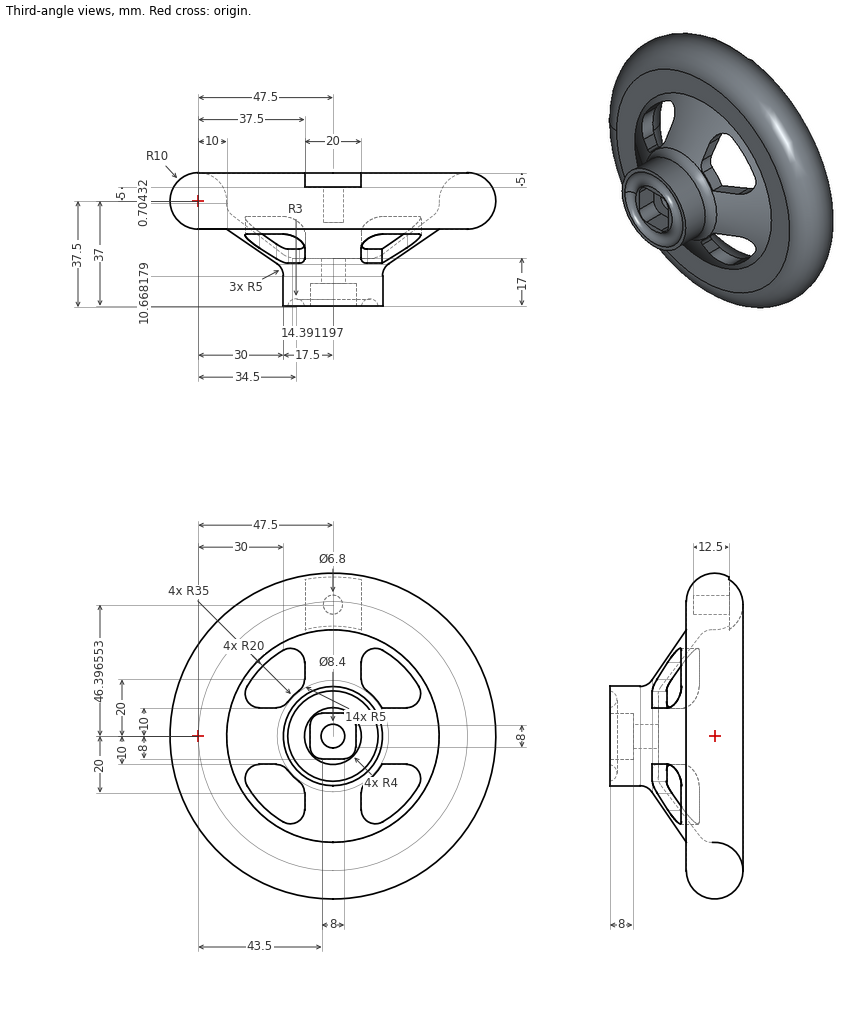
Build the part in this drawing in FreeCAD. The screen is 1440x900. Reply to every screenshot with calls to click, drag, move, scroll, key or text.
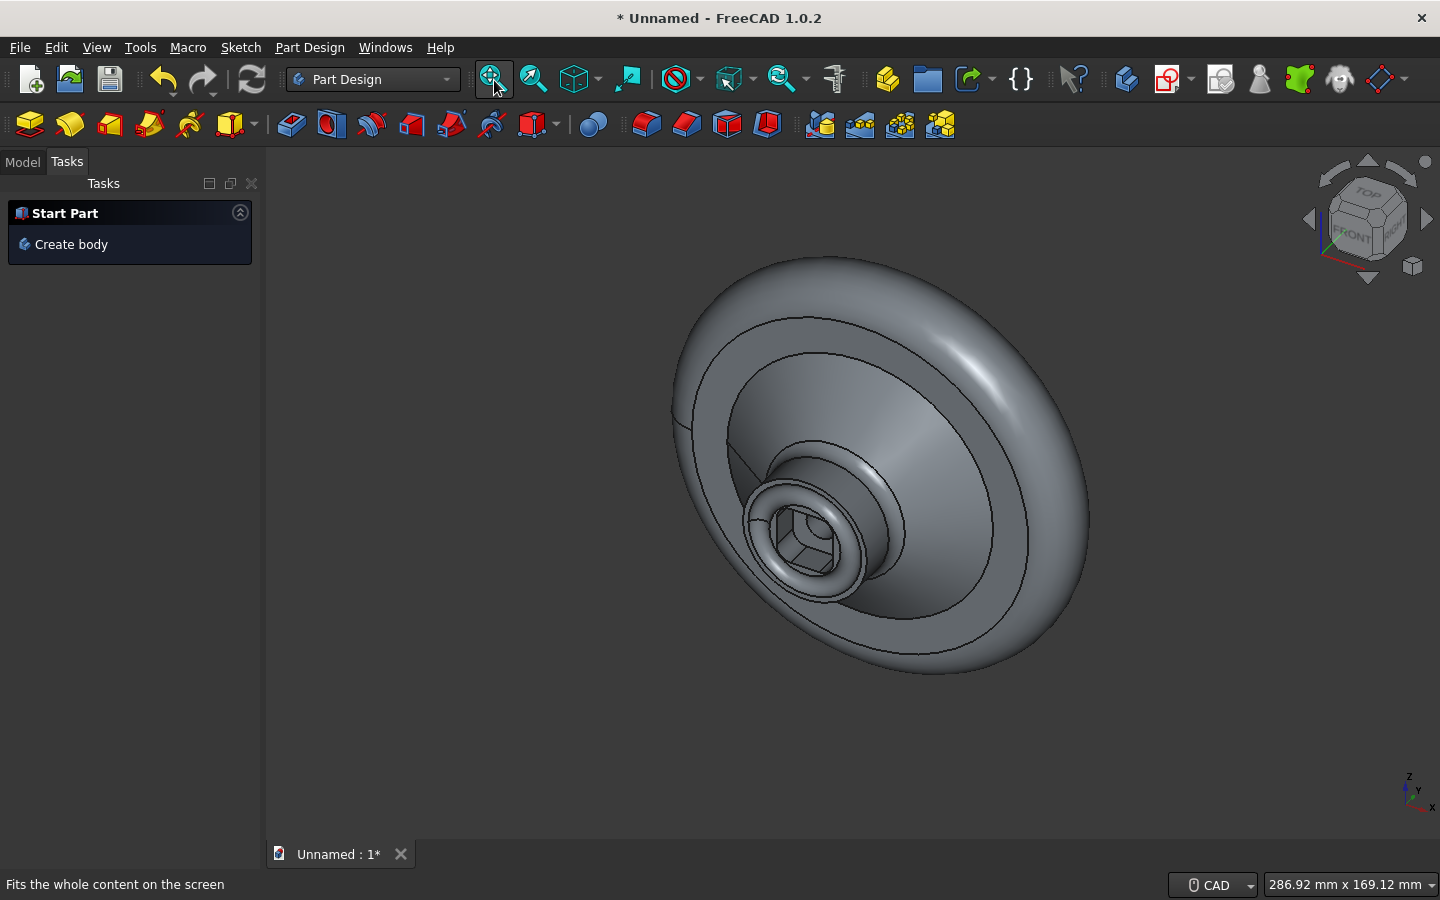
click(1168, 80)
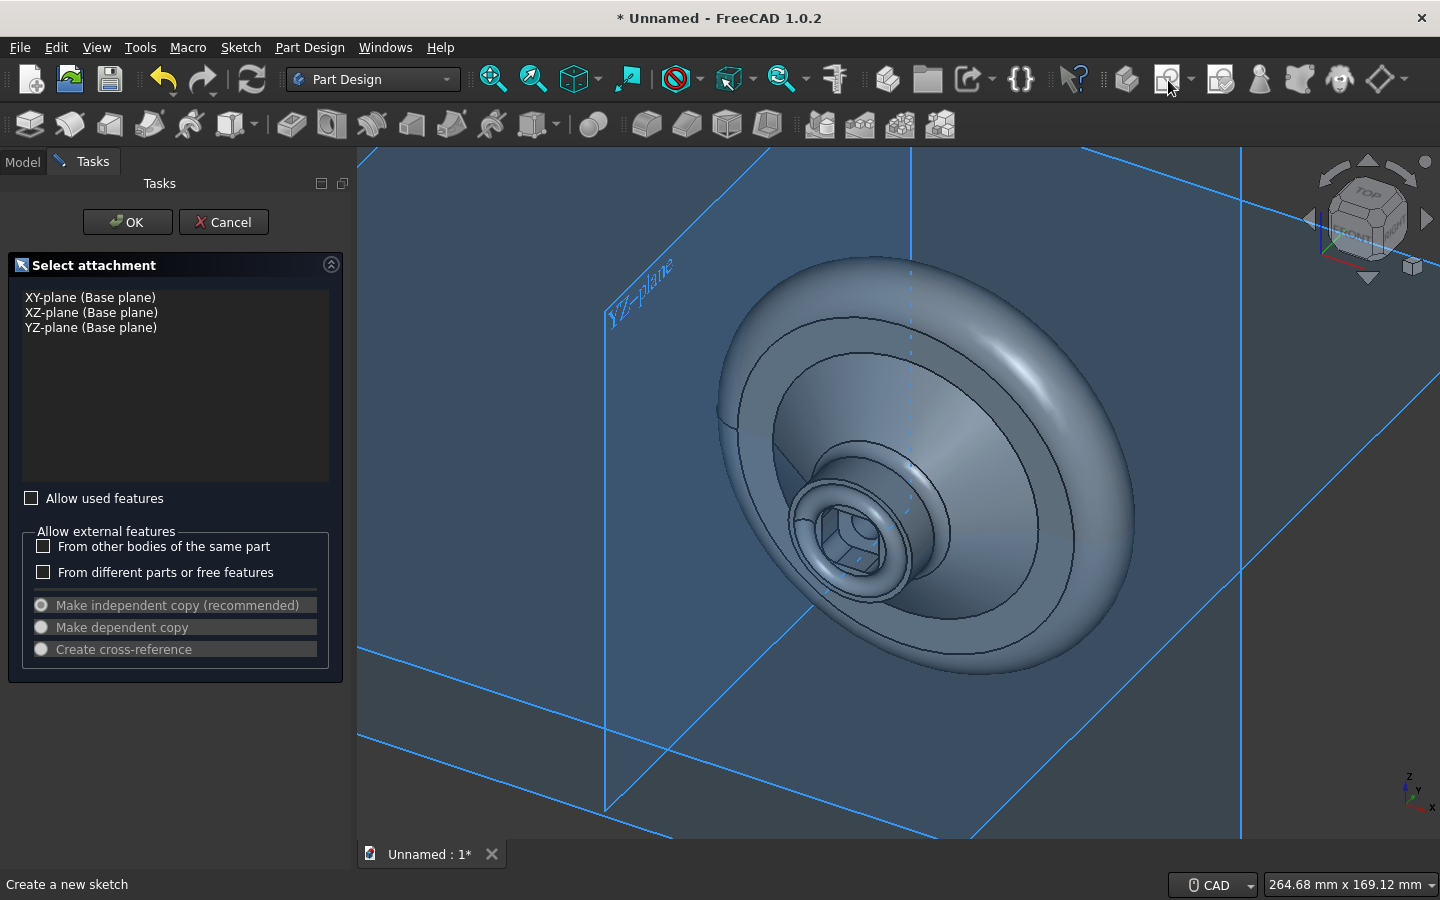
click(82, 298)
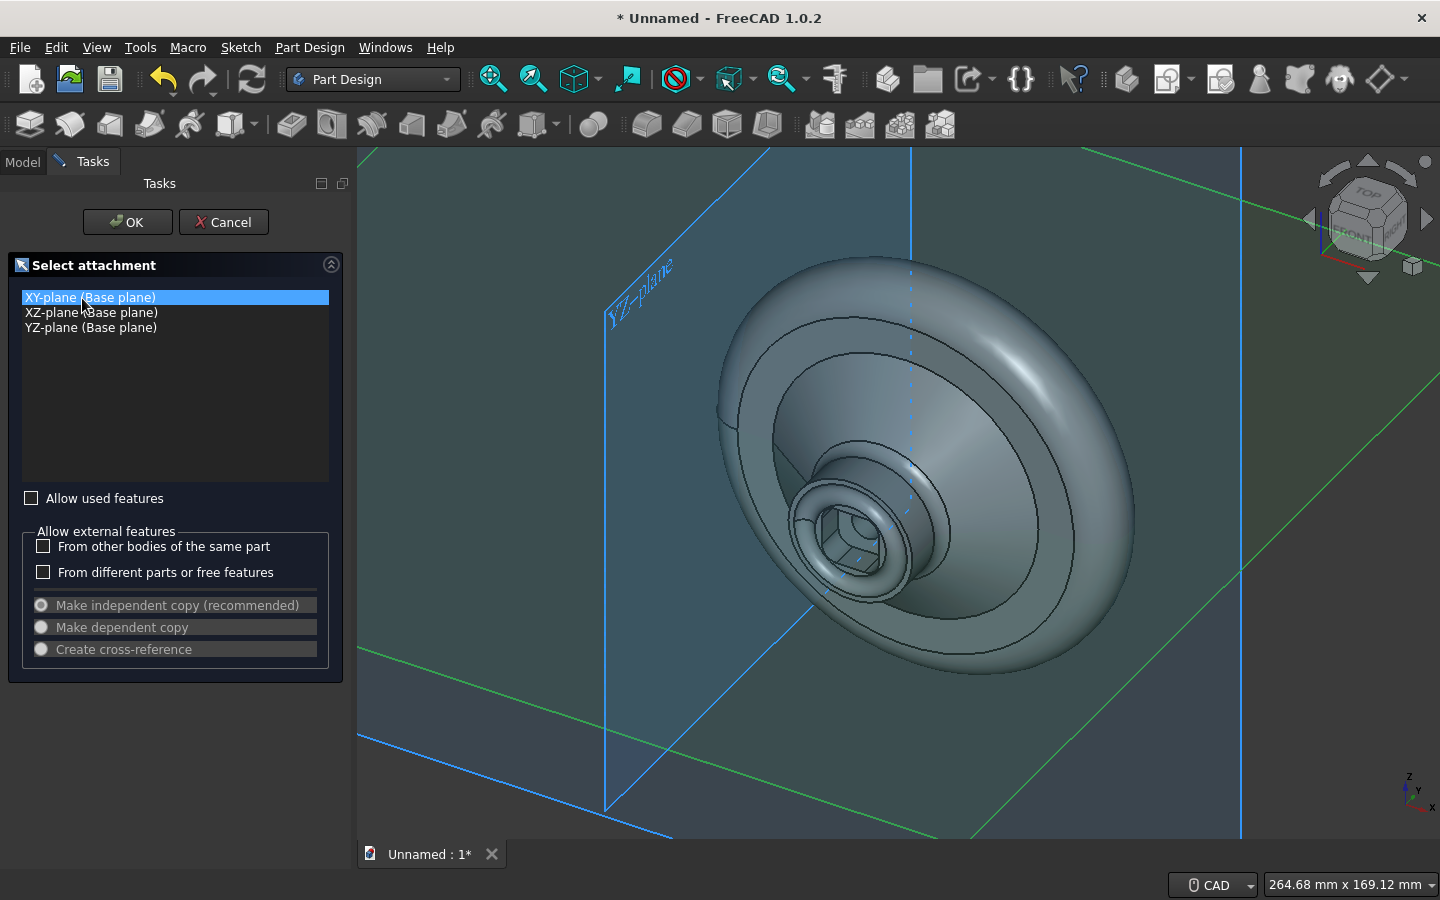
click(128, 222)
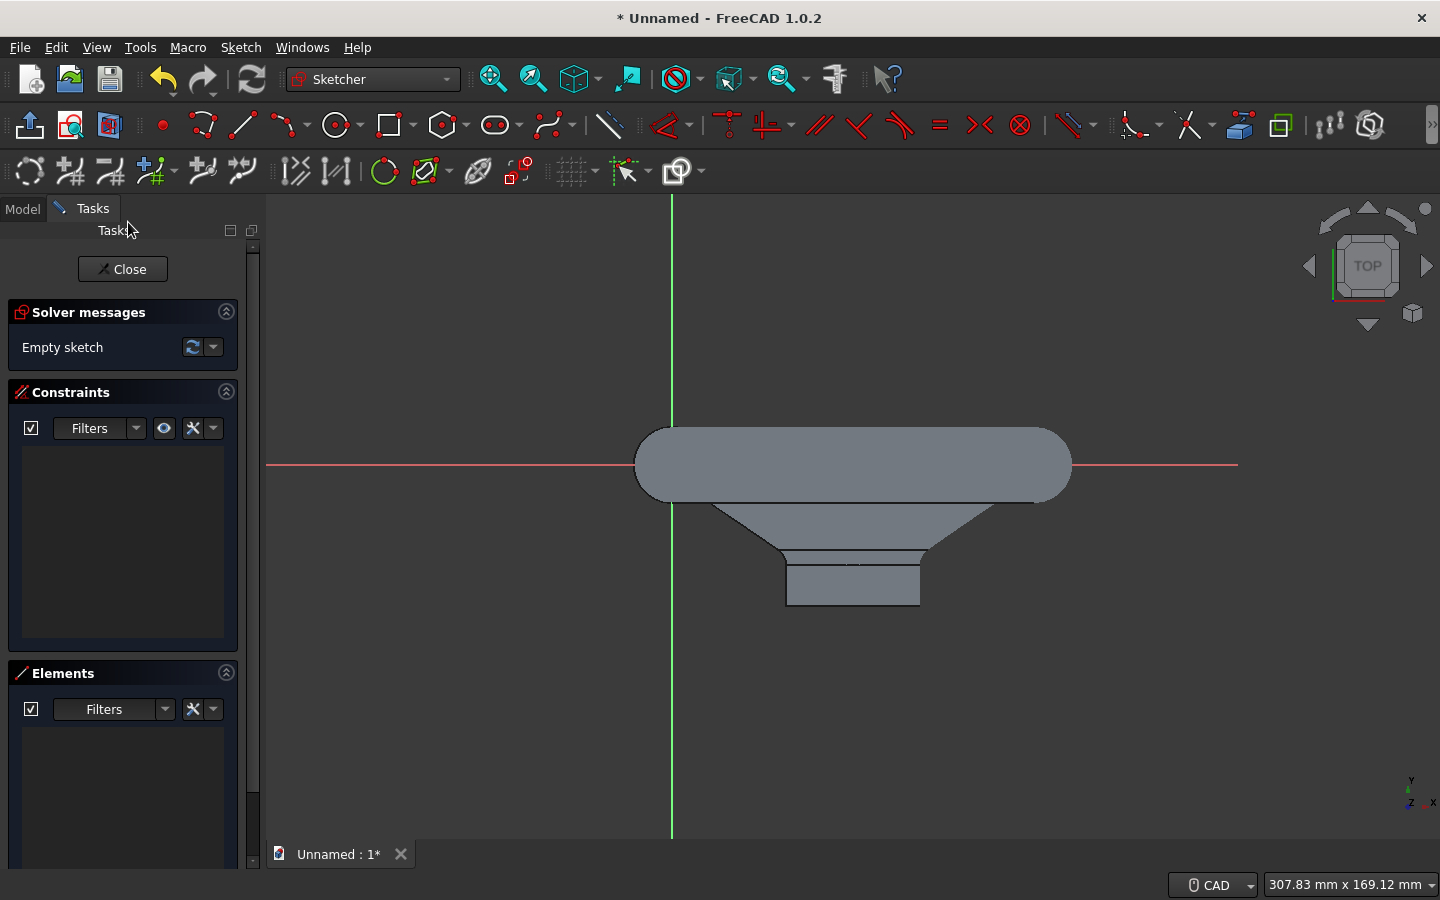
click(110, 126)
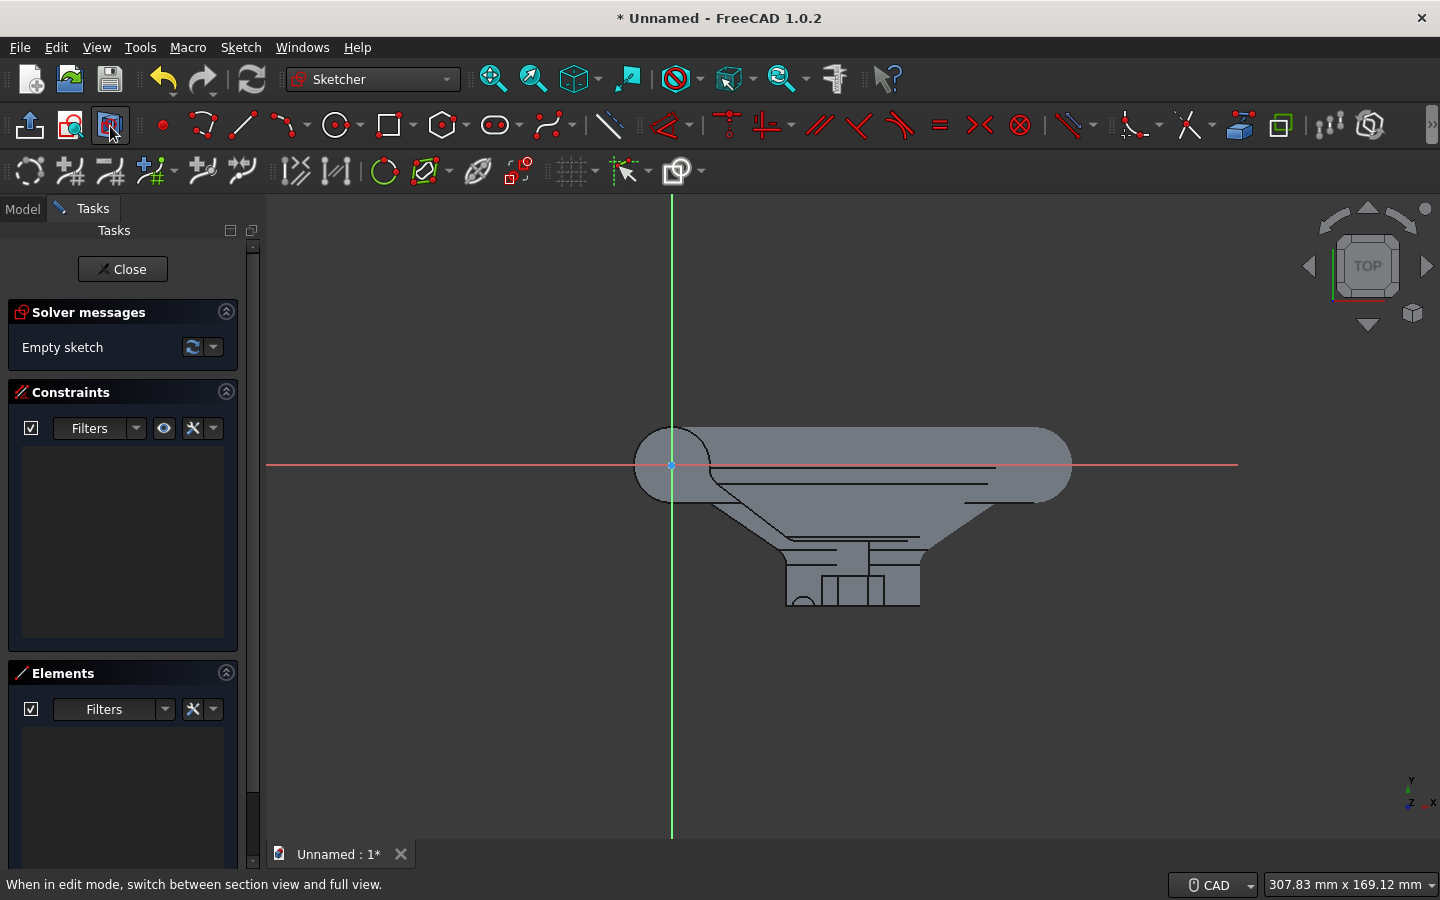
scroll(862, 426, up, 11)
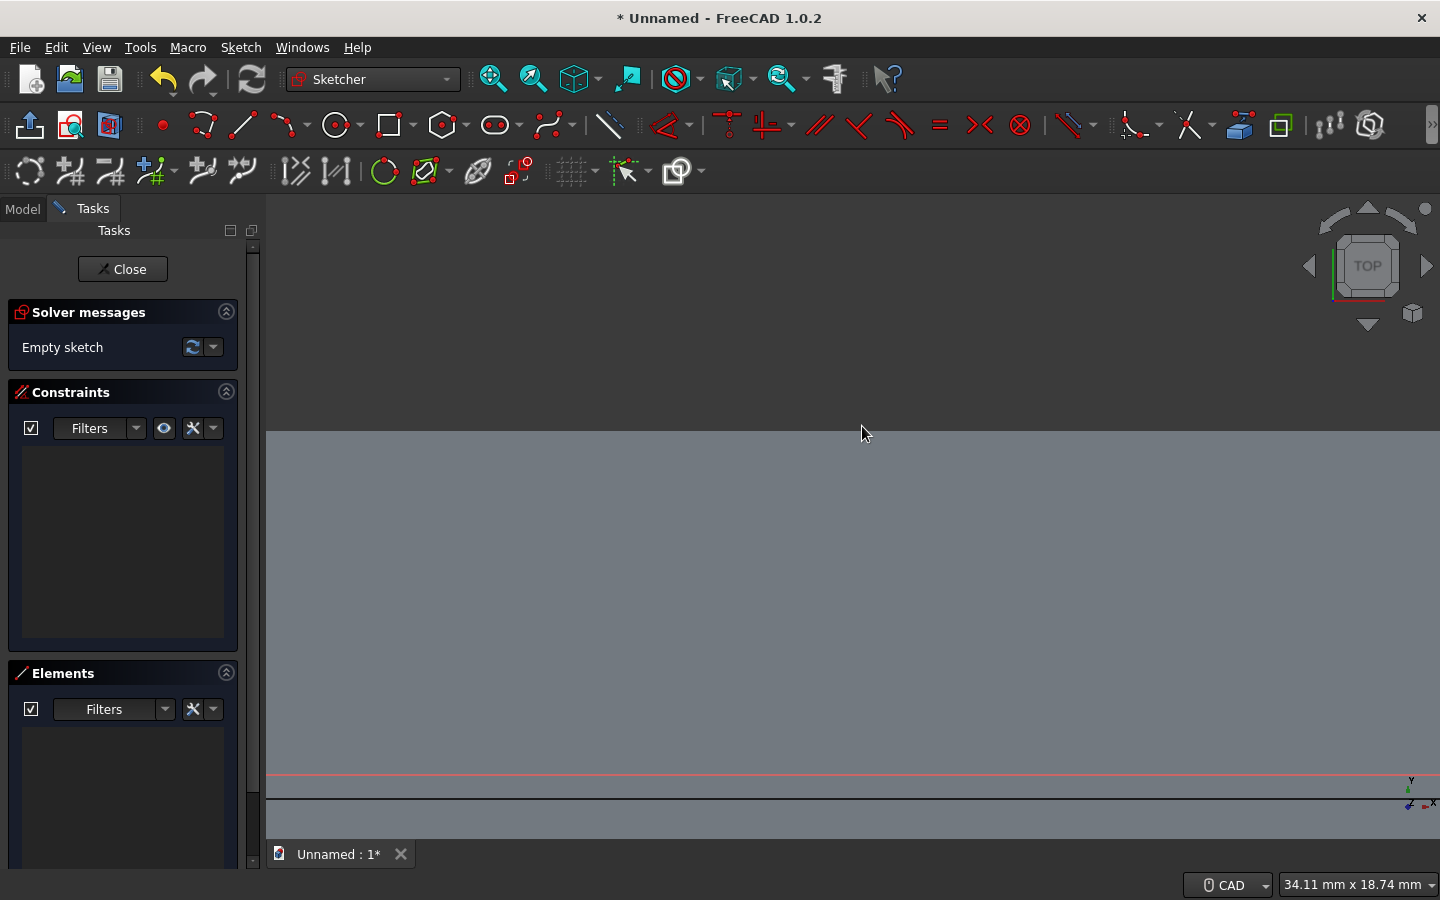
click(390, 126)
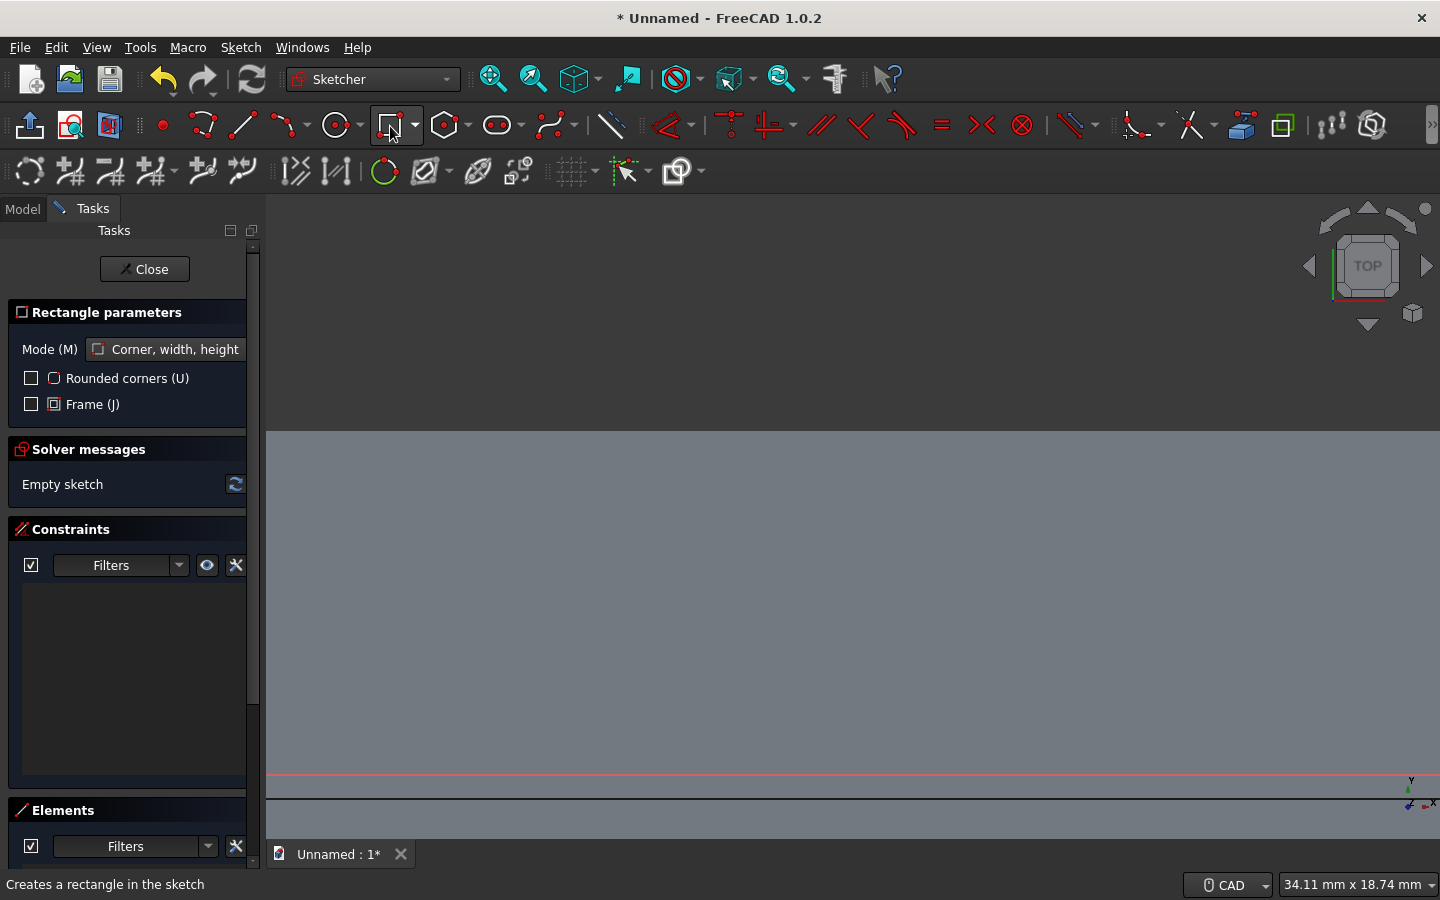
click(433, 431)
move(1121, 603)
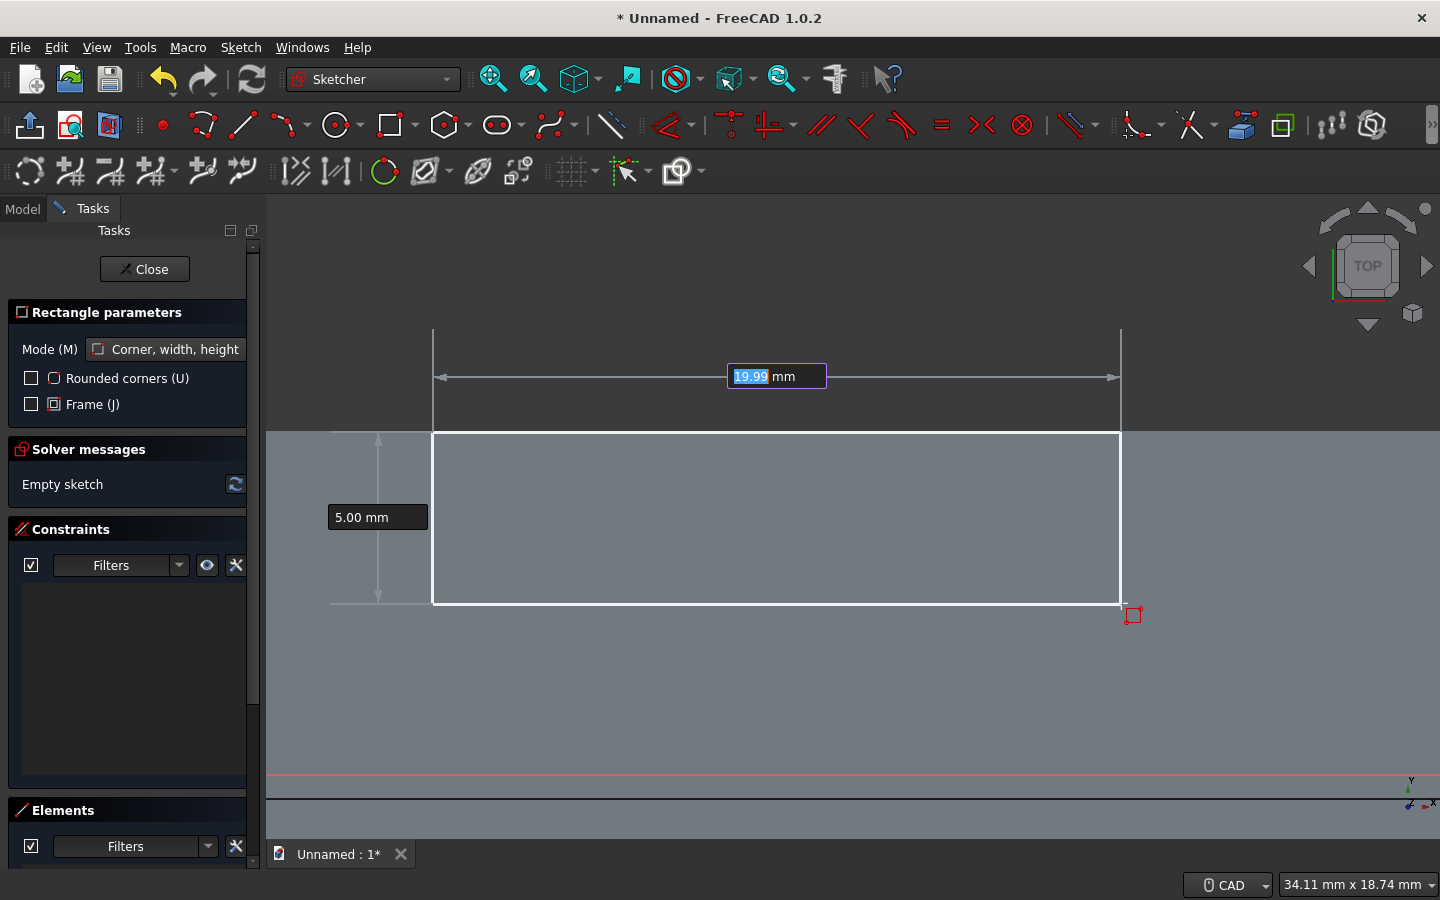
text(20)
key(Tab)
text(5)
key(Return)
key(Escape)